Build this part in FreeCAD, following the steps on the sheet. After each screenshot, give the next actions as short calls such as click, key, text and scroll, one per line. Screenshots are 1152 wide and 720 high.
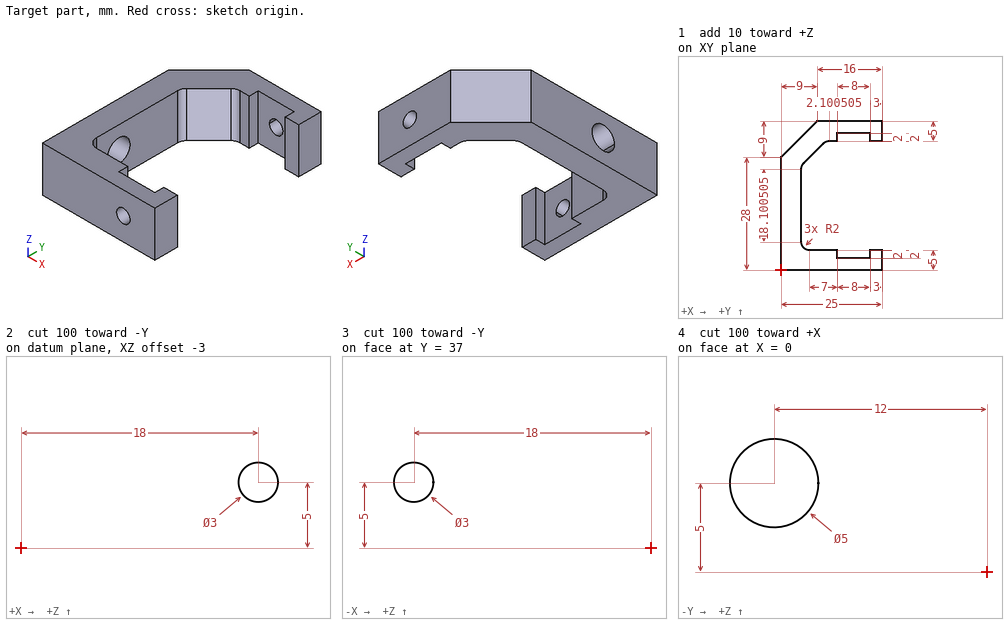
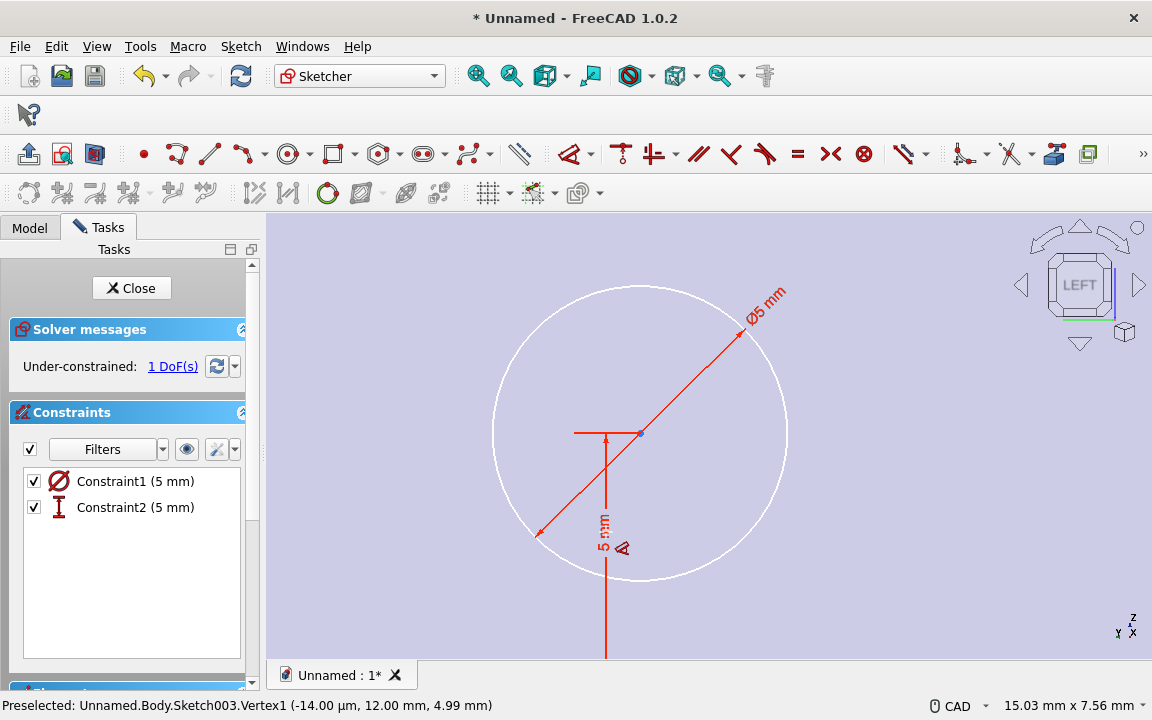
click(640, 433)
click(813, 399)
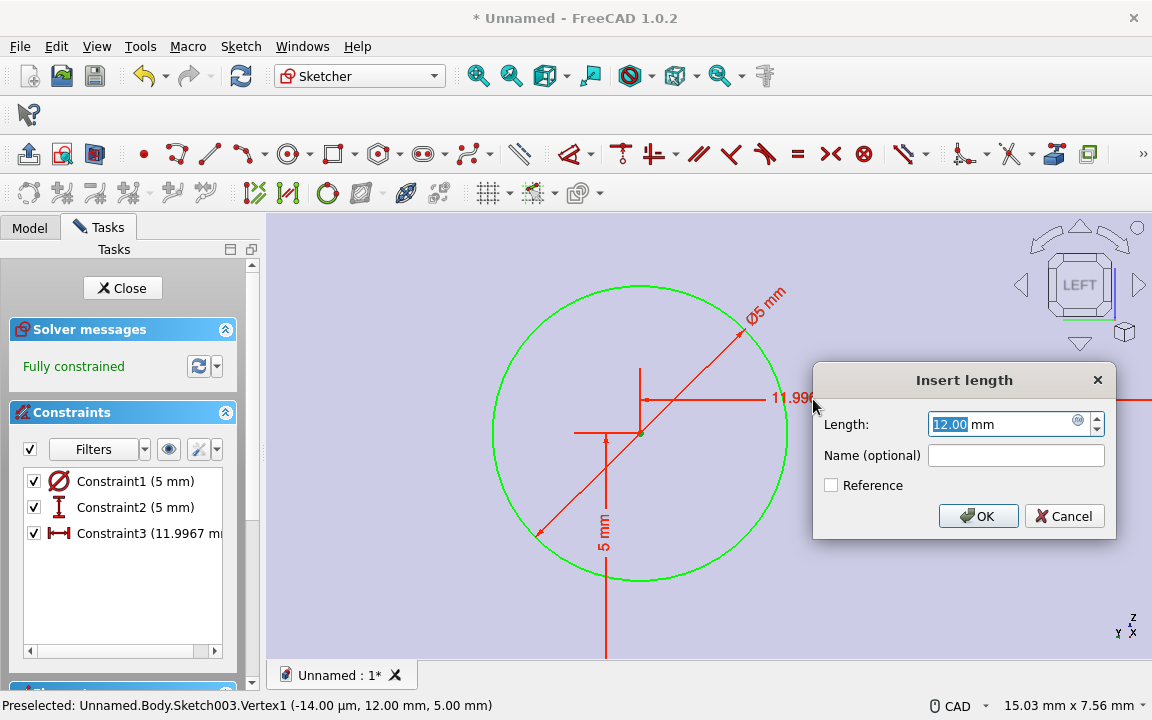
text(12)
key(Return)
key(Escape)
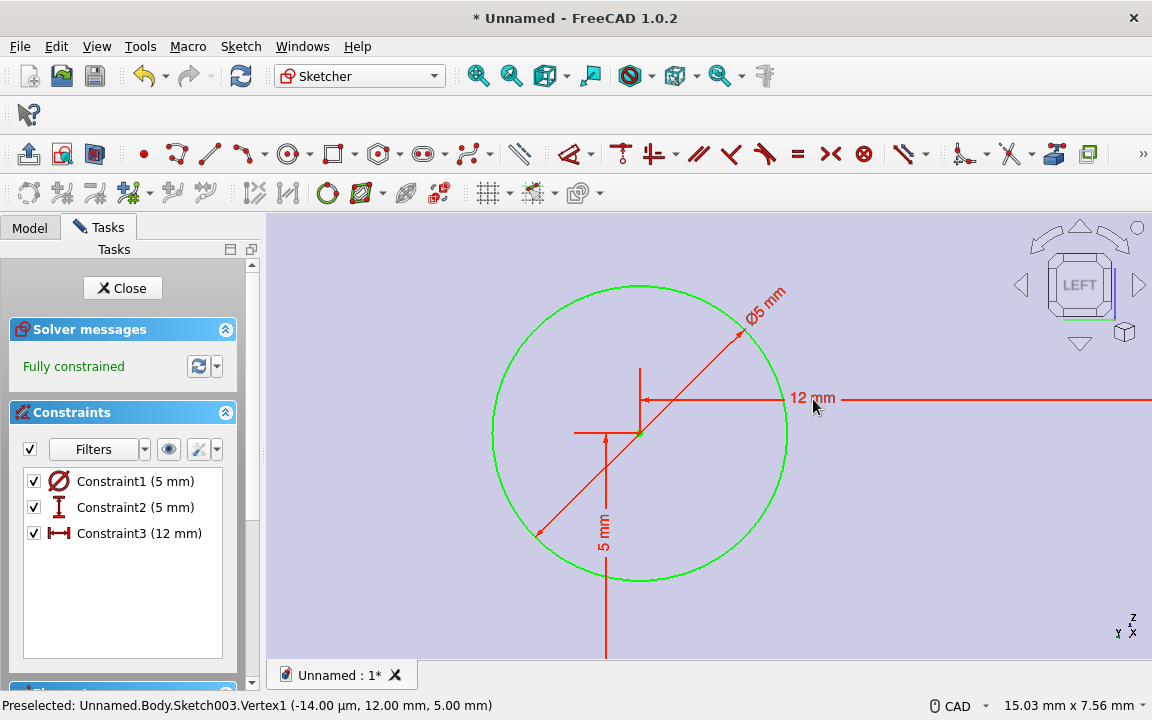
click(123, 288)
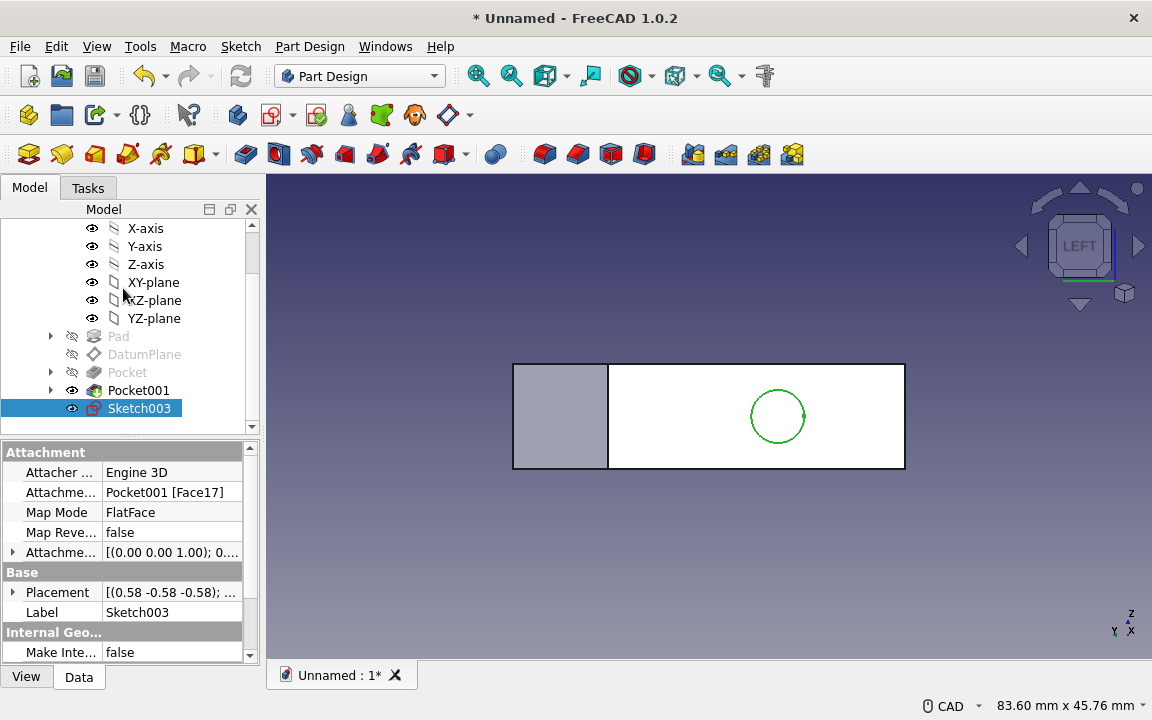
click(246, 154)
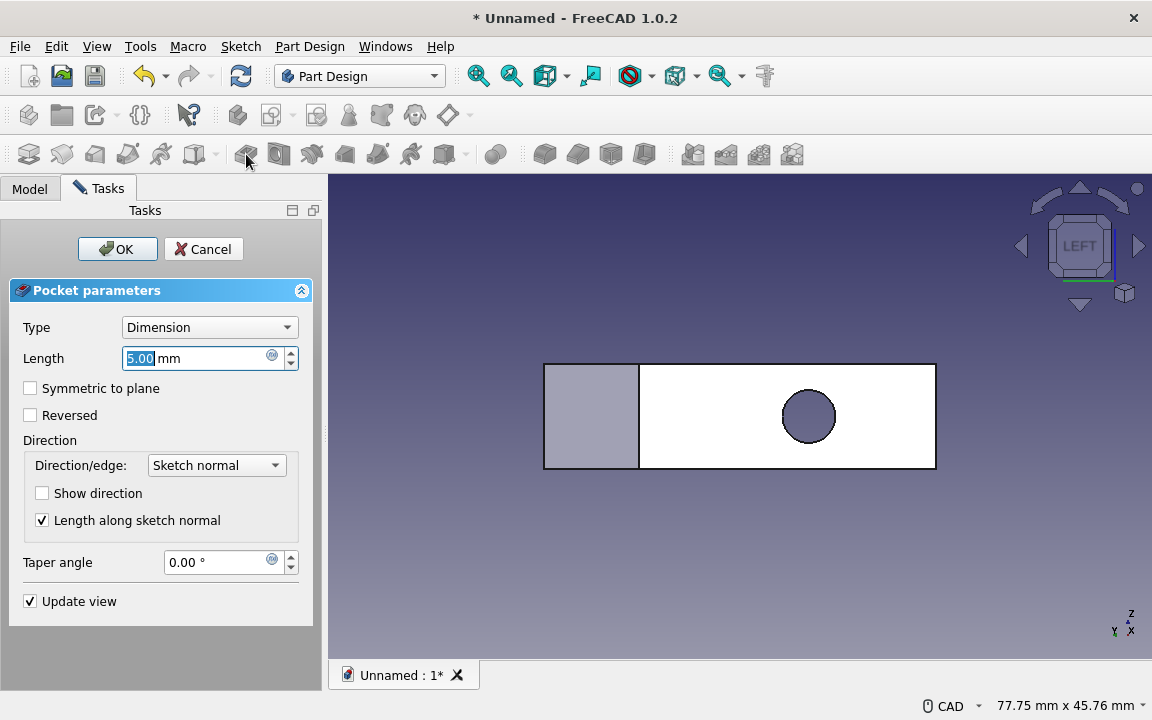
text(100)
key(Tab)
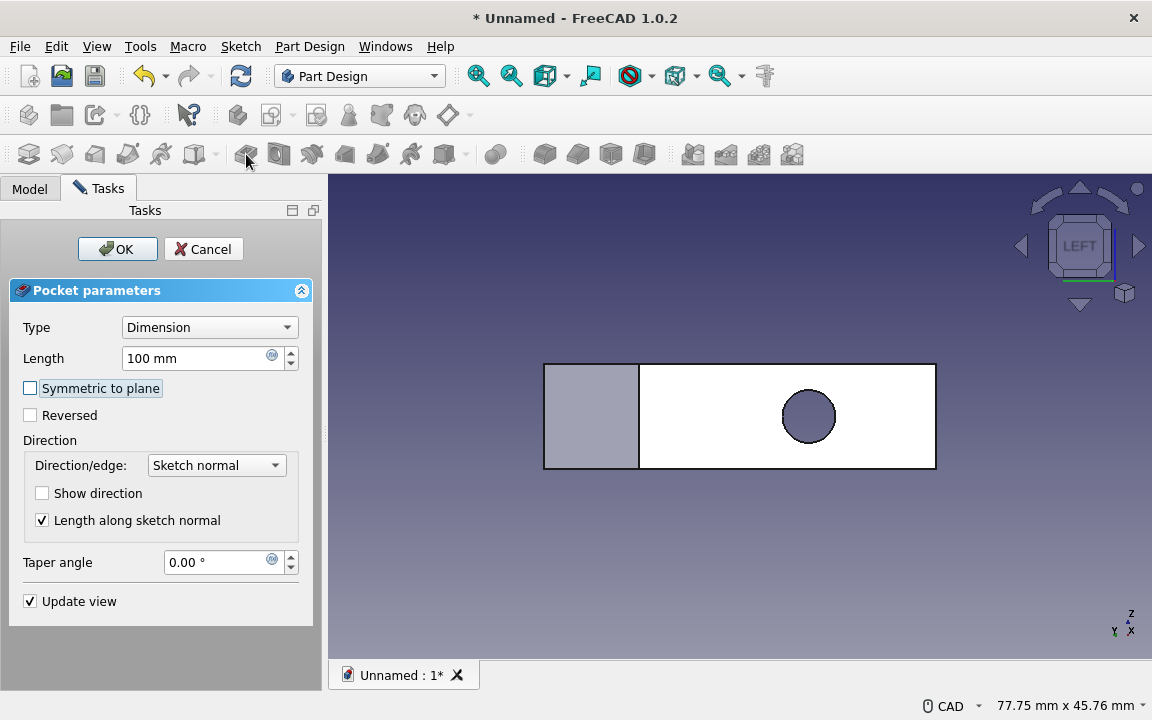
click(118, 249)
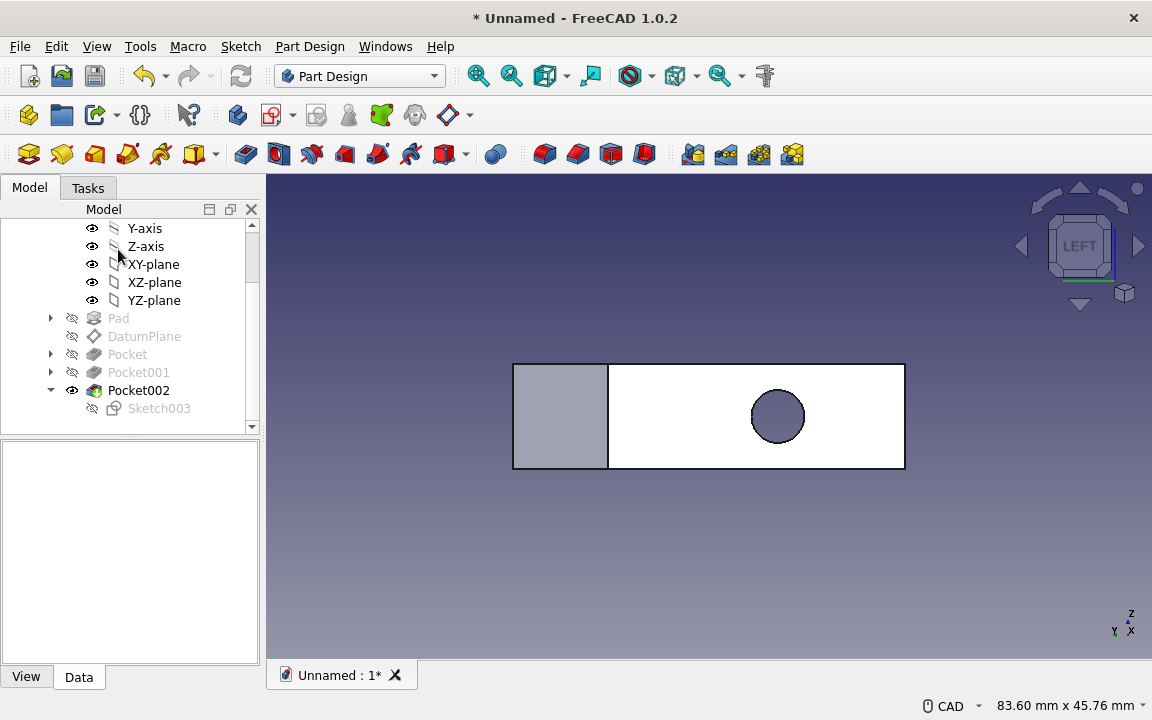
key(0)